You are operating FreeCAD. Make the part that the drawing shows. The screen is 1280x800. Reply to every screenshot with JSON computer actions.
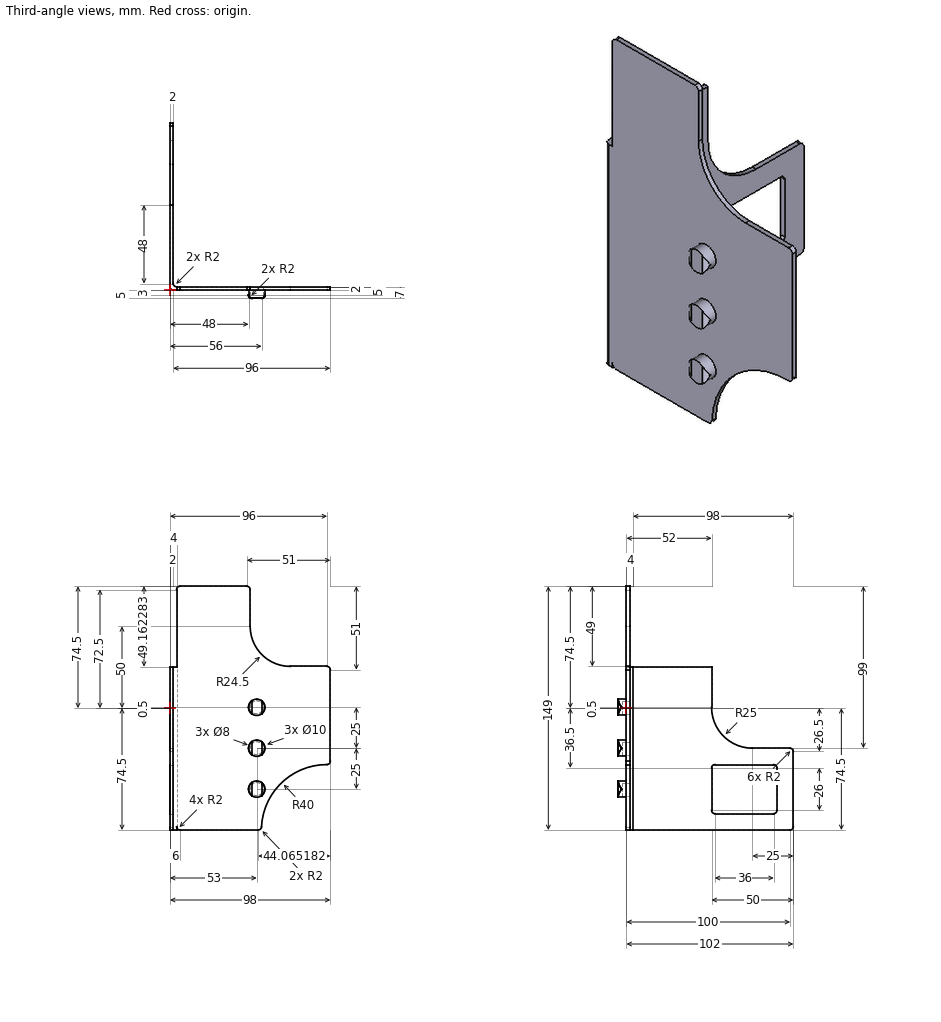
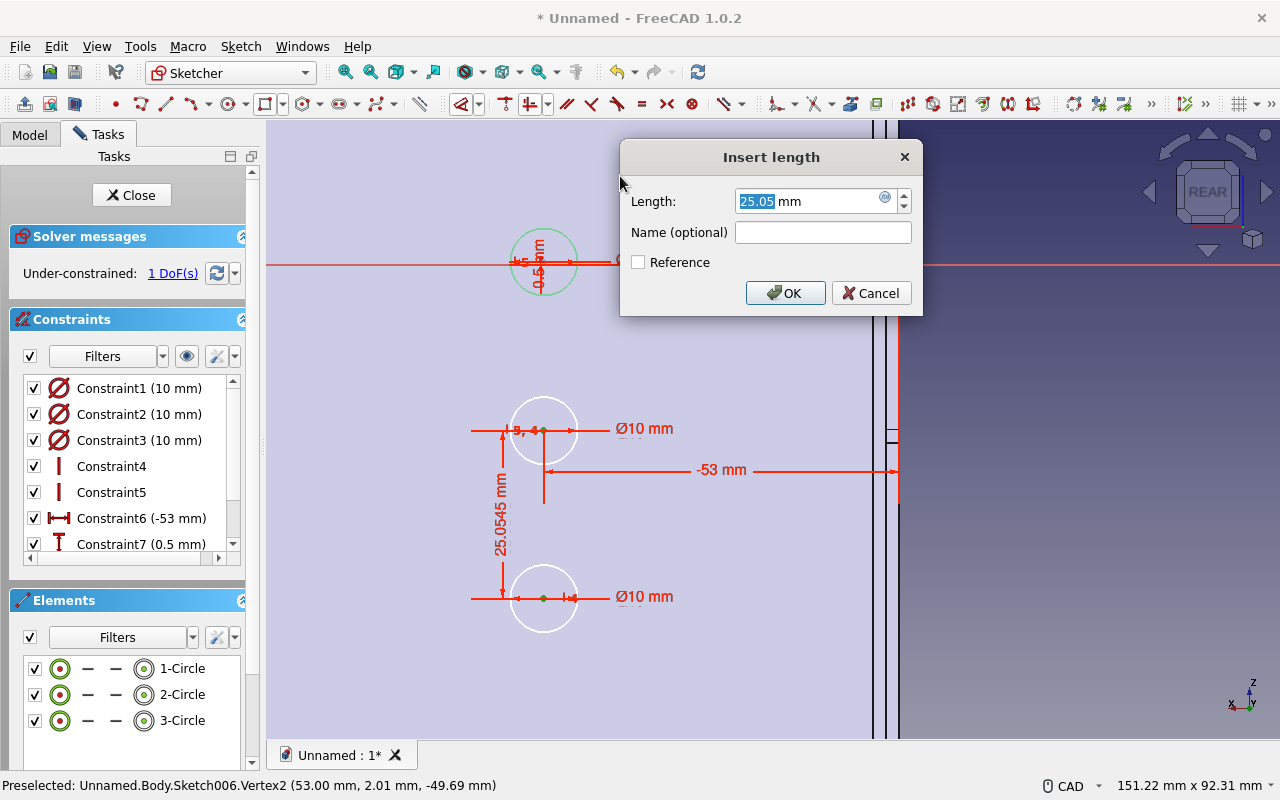
{"action": "type", "text": "25"}
{"action": "key", "text": "Return"}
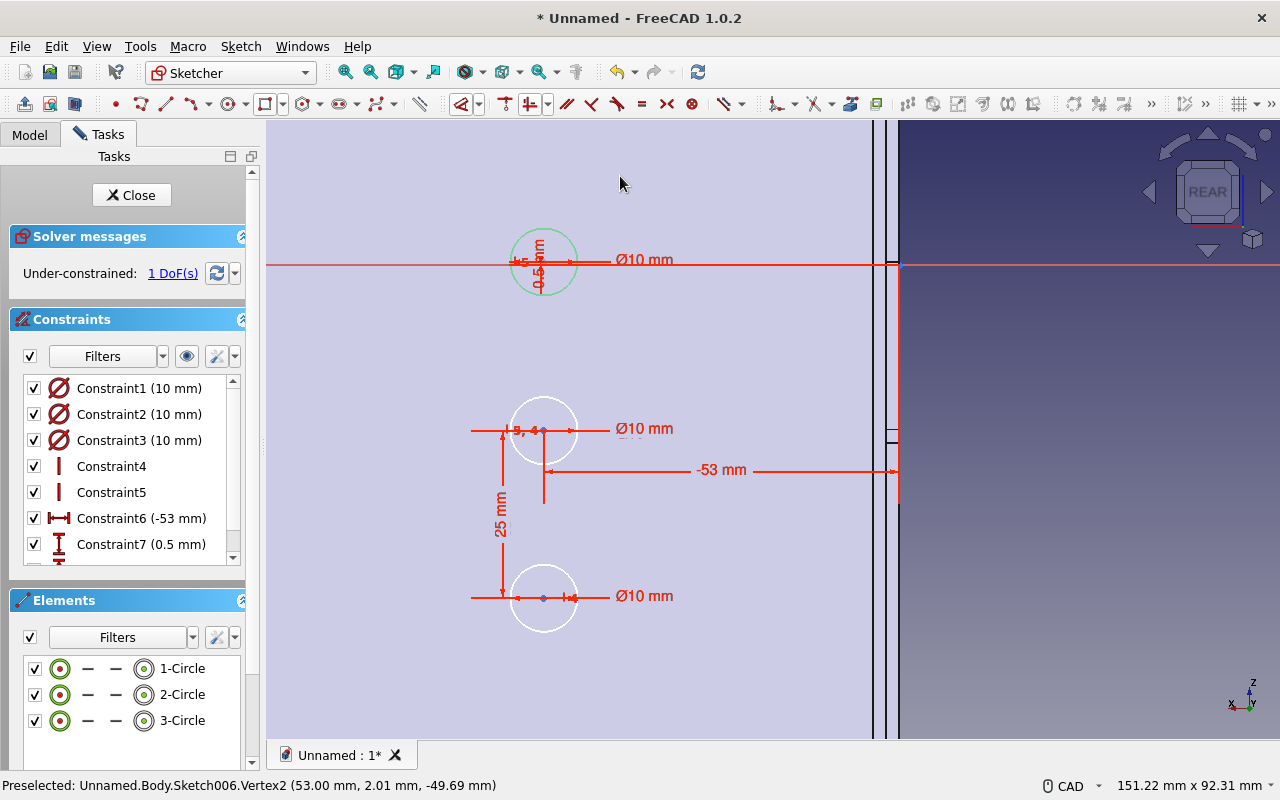
{"action": "left_click", "coordinate": [544, 431]}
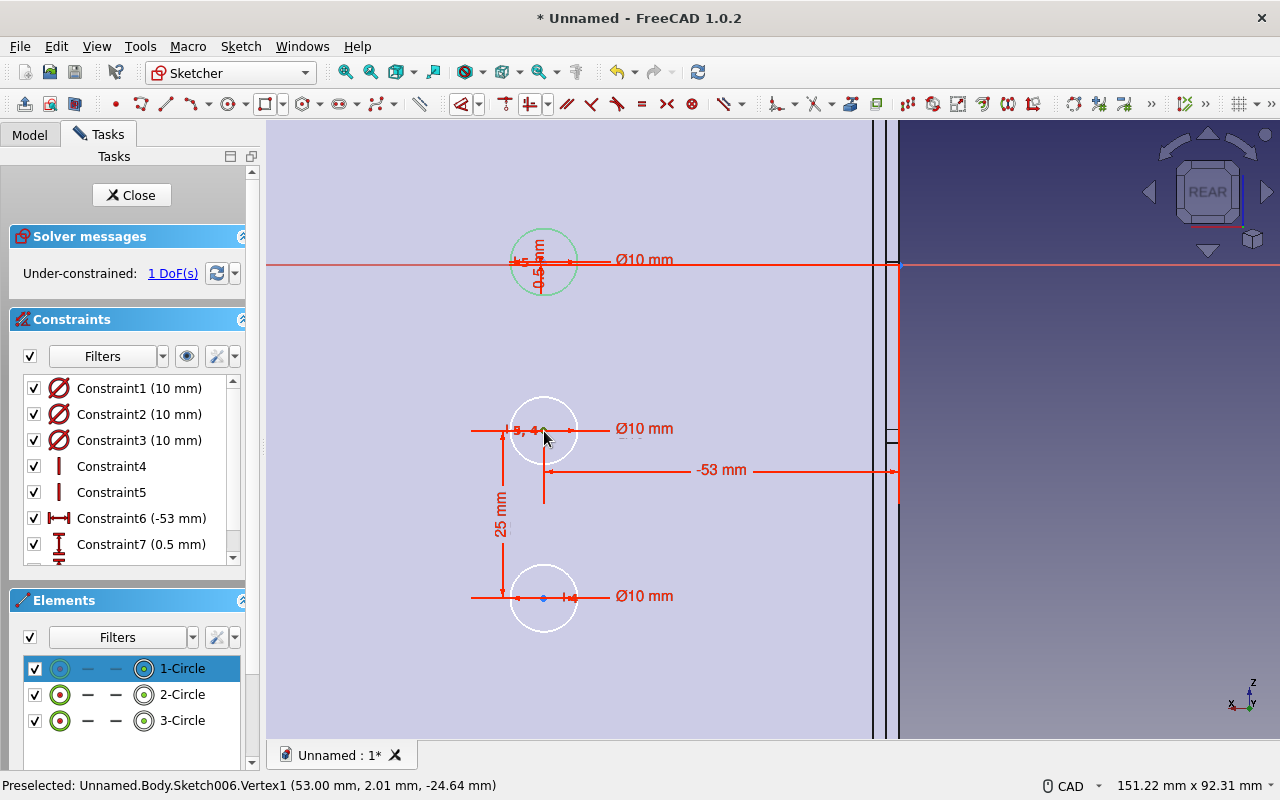
{"action": "left_click", "coordinate": [544, 262]}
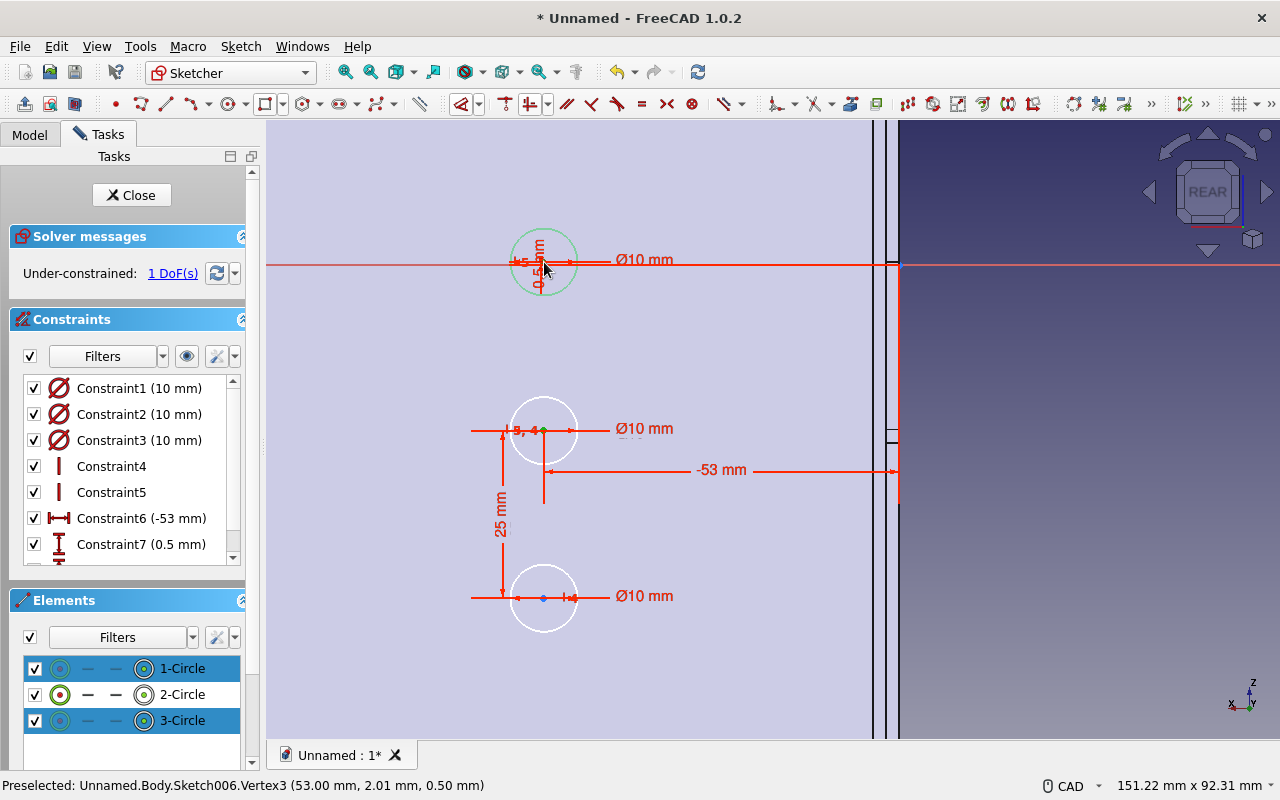
{"action": "left_click", "coordinate": [478, 104]}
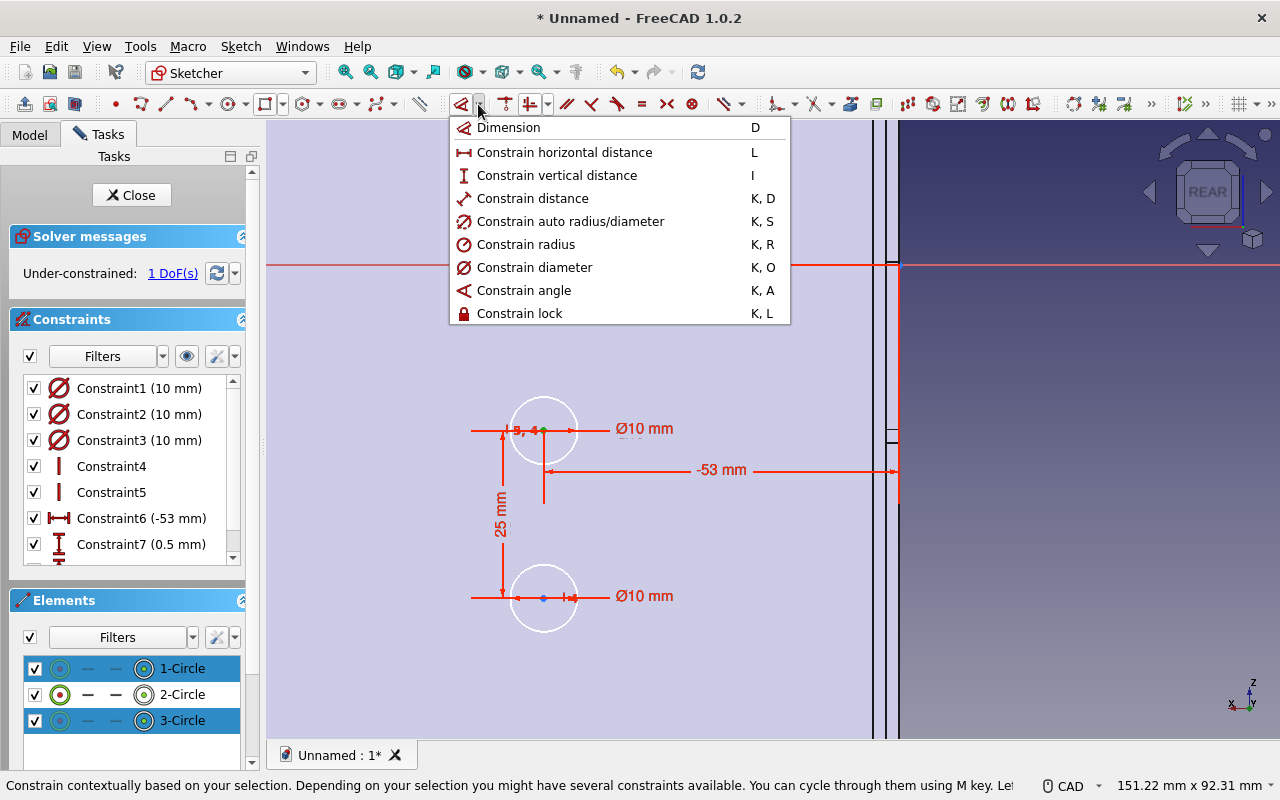
{"action": "left_click", "coordinate": [620, 176]}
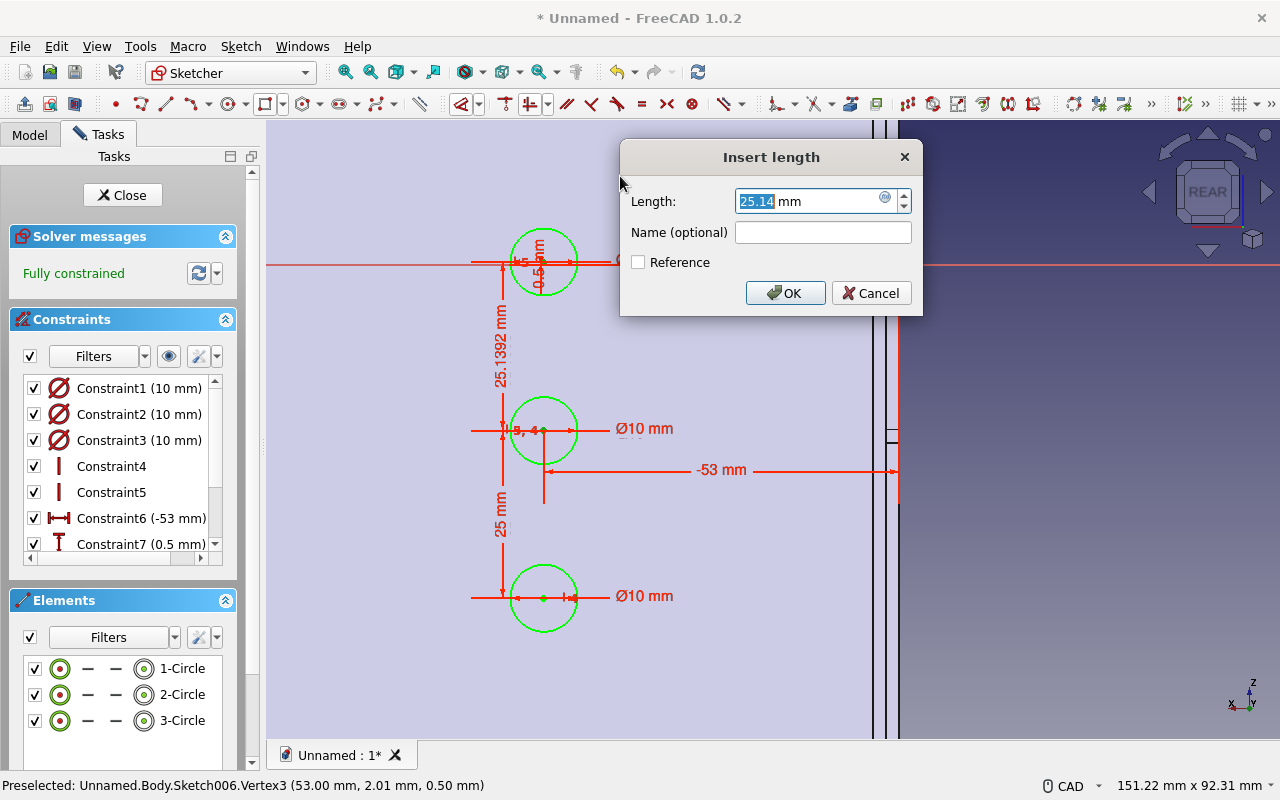
{"action": "type", "text": "25"}
{"action": "key", "text": "Return"}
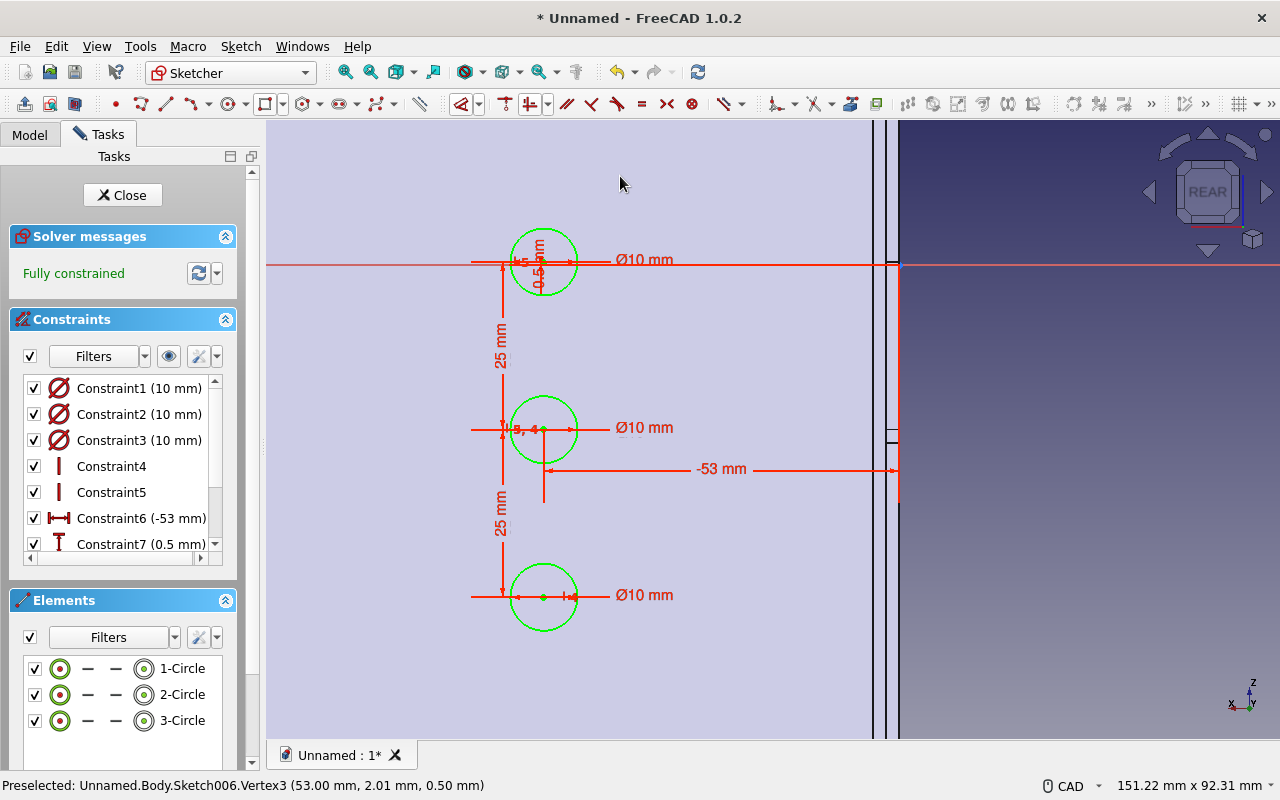
{"action": "left_click", "coordinate": [123, 195]}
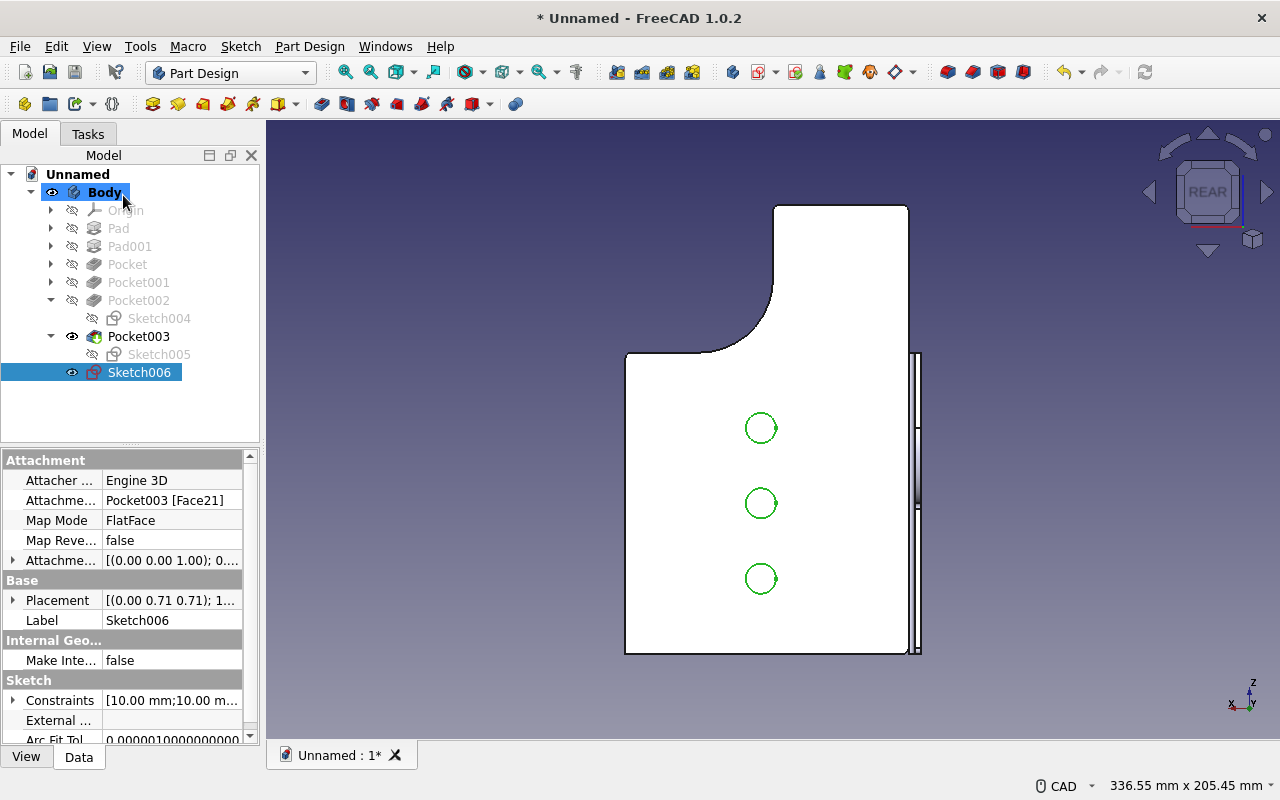
{"action": "left_click", "coordinate": [153, 104]}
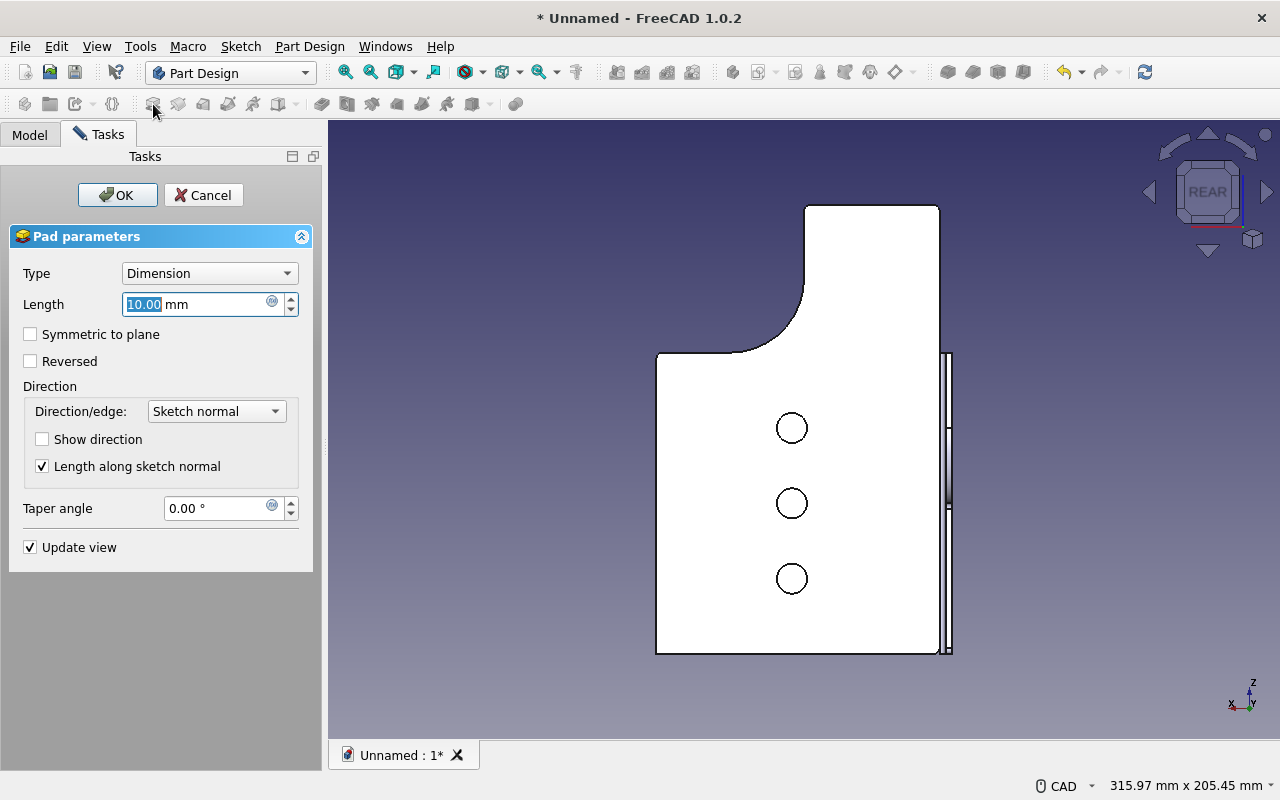
{"action": "type", "text": "7"}
{"action": "key", "text": "Tab"}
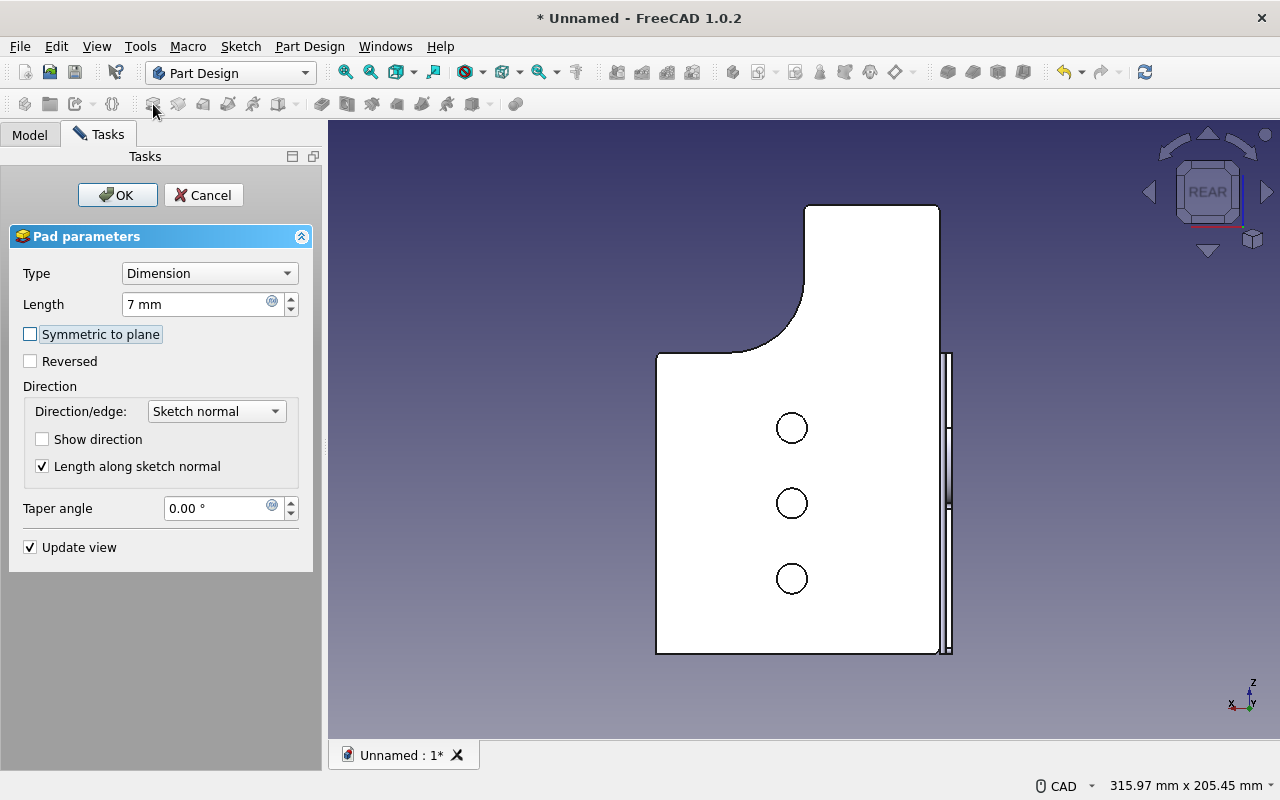
{"action": "left_click", "coordinate": [31, 361]}